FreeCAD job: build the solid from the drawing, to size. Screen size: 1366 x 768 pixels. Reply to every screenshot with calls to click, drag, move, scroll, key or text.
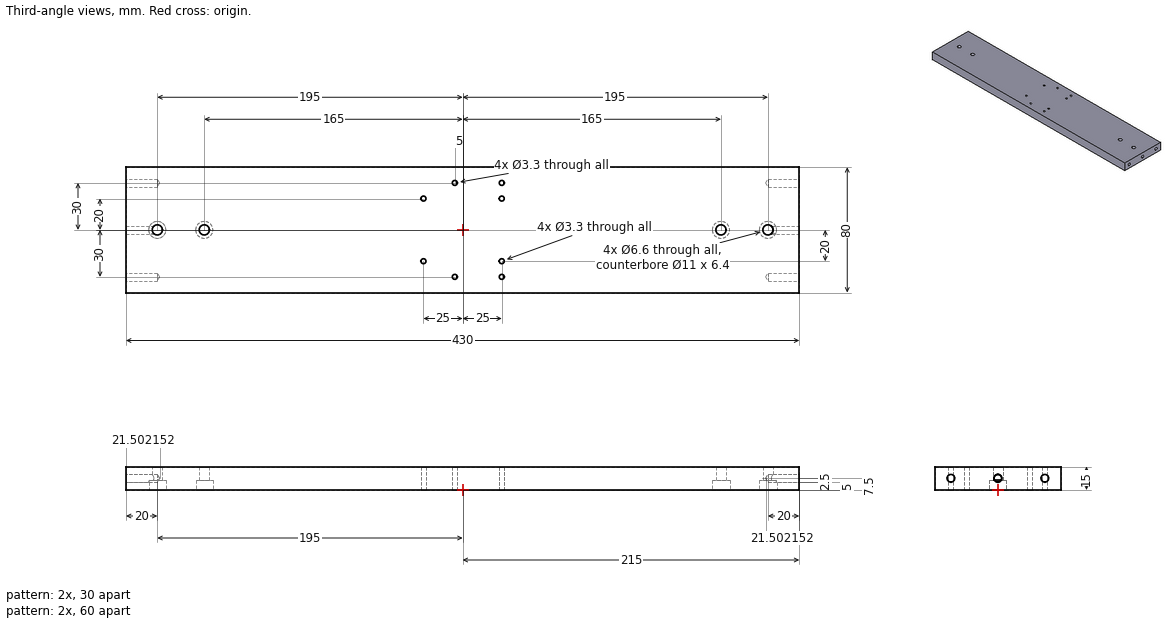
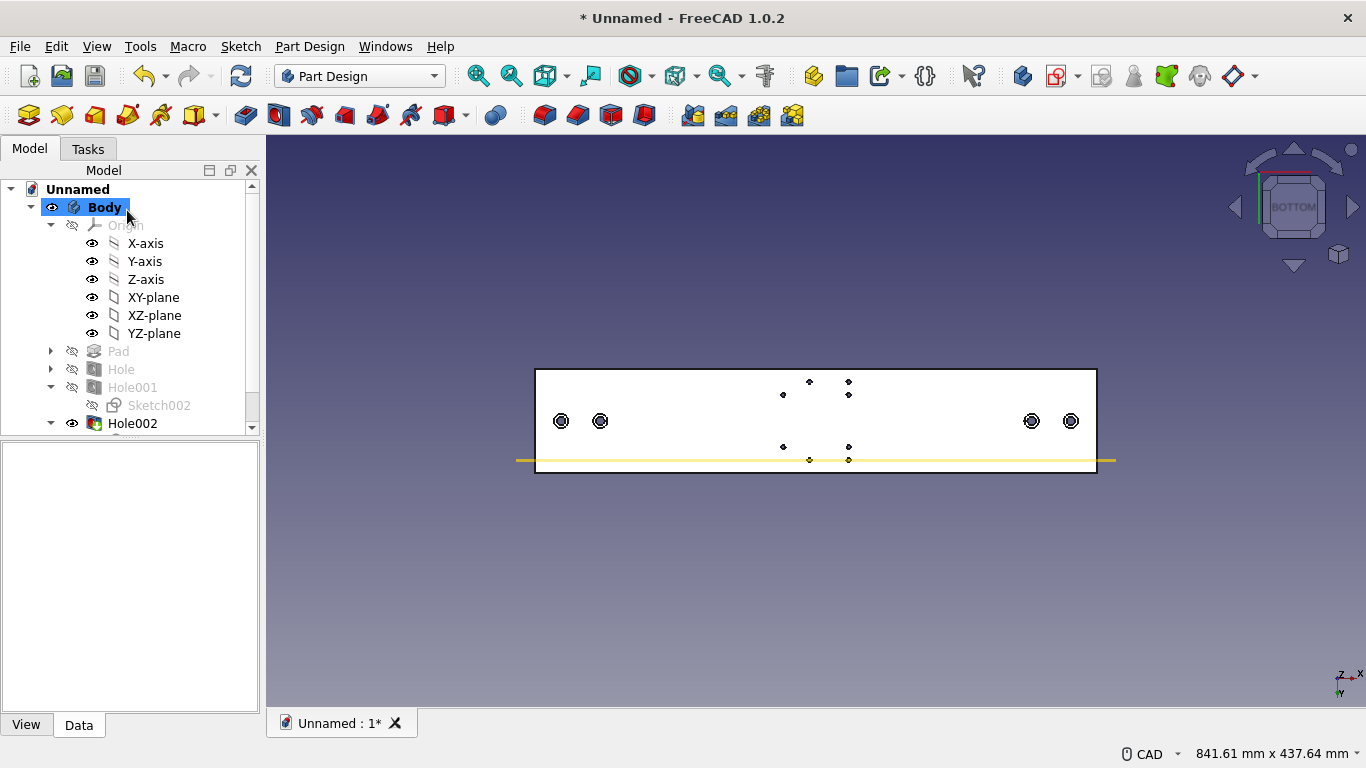
scroll(101, 311, down, 3)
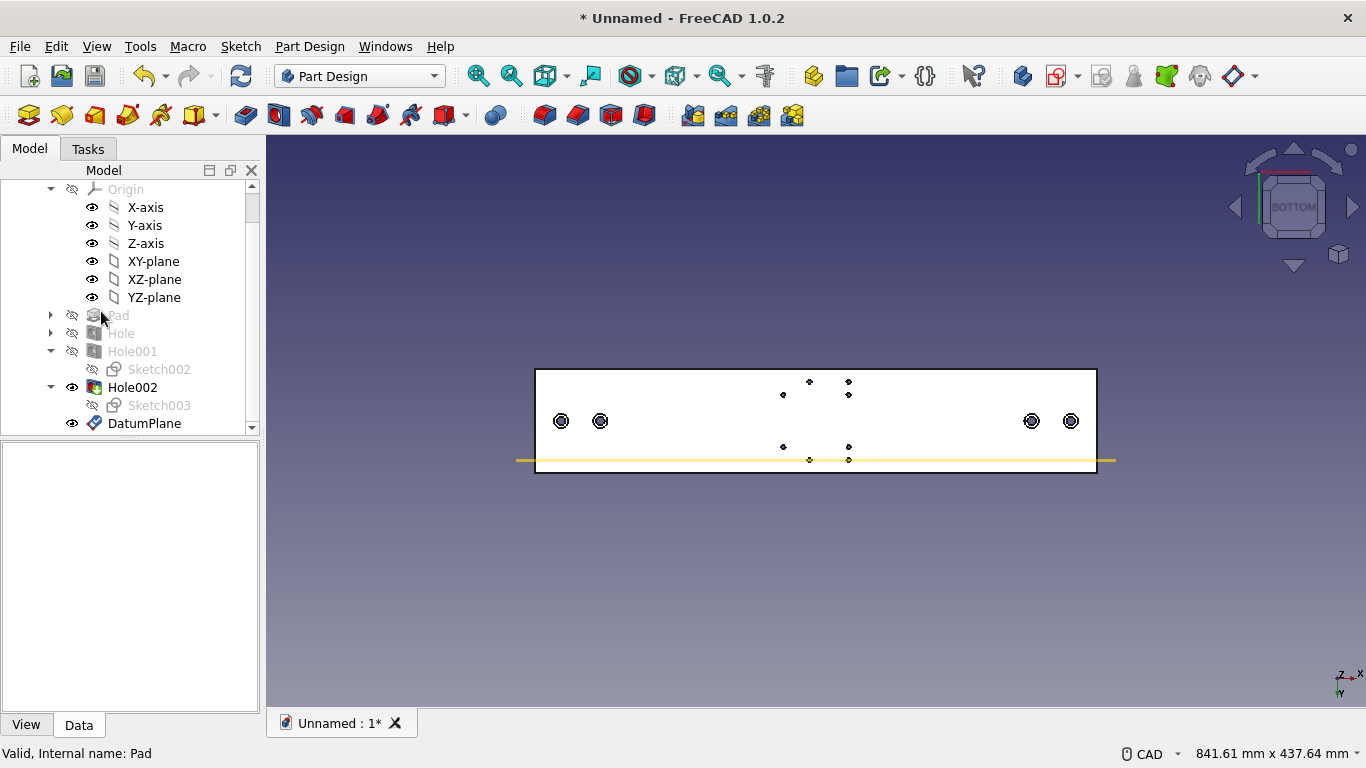
click(117, 423)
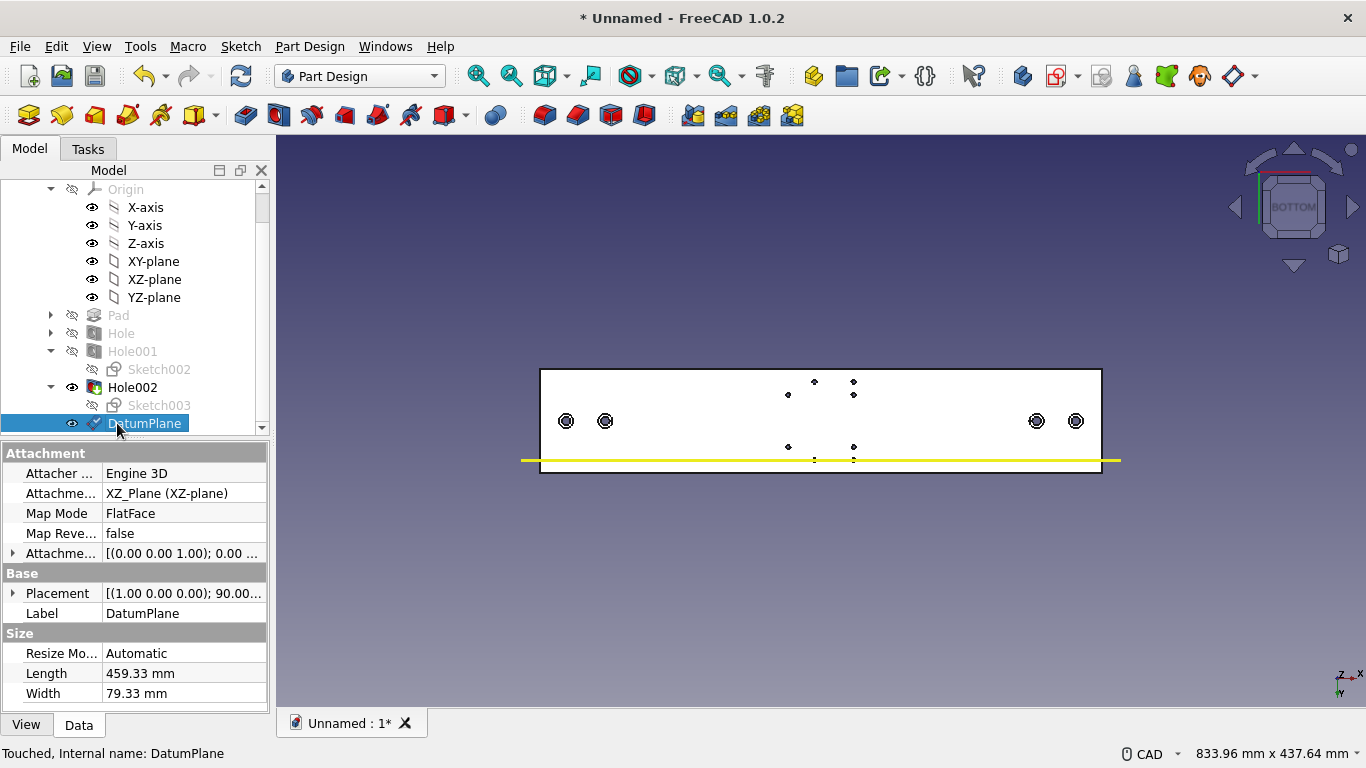
click(1056, 76)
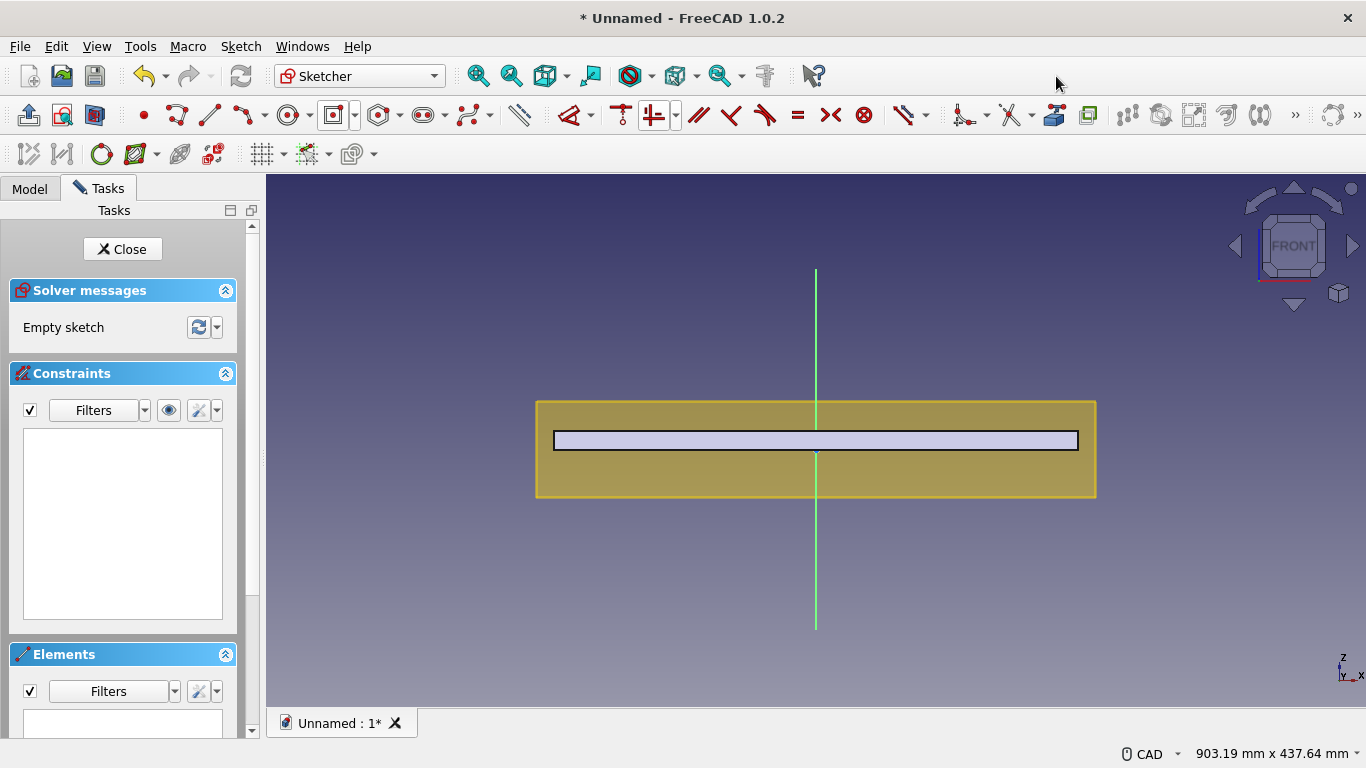
click(95, 116)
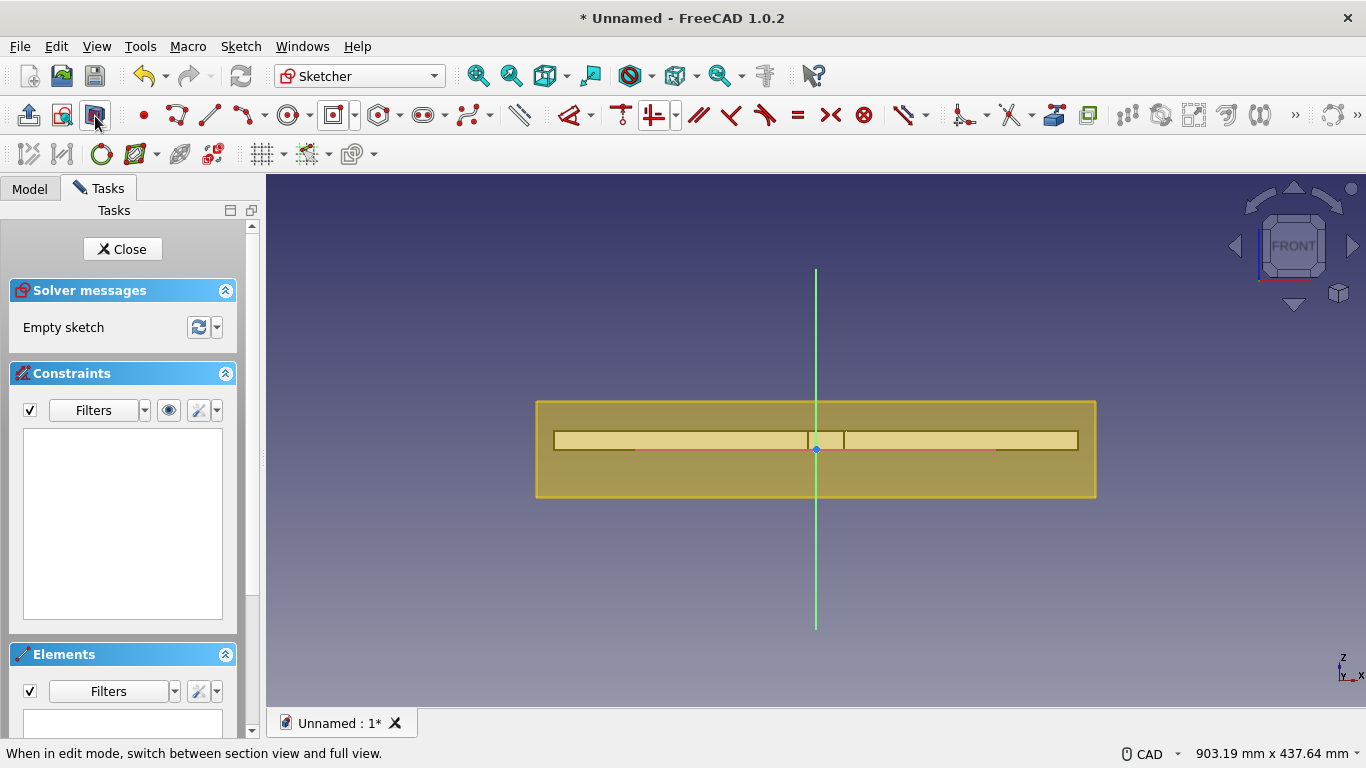
scroll(1080, 442, up, 14)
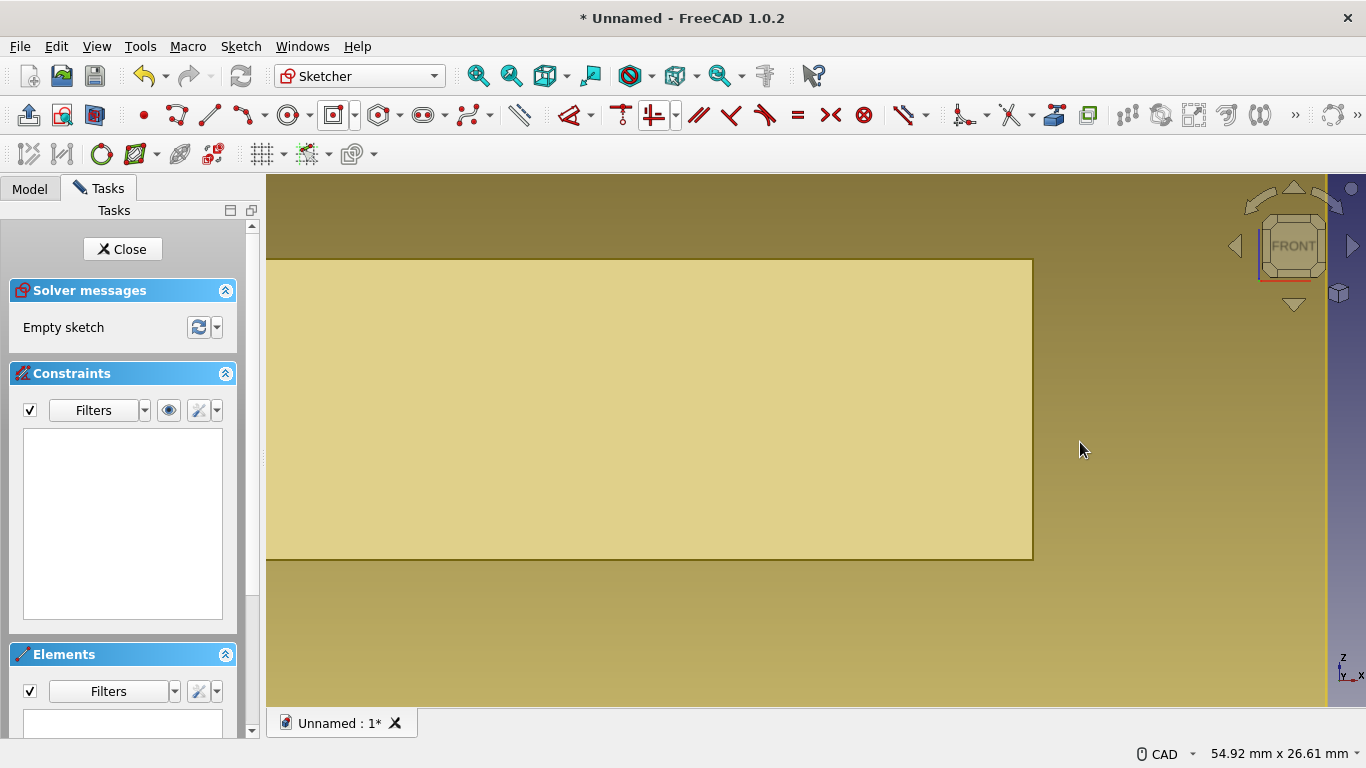
click(177, 116)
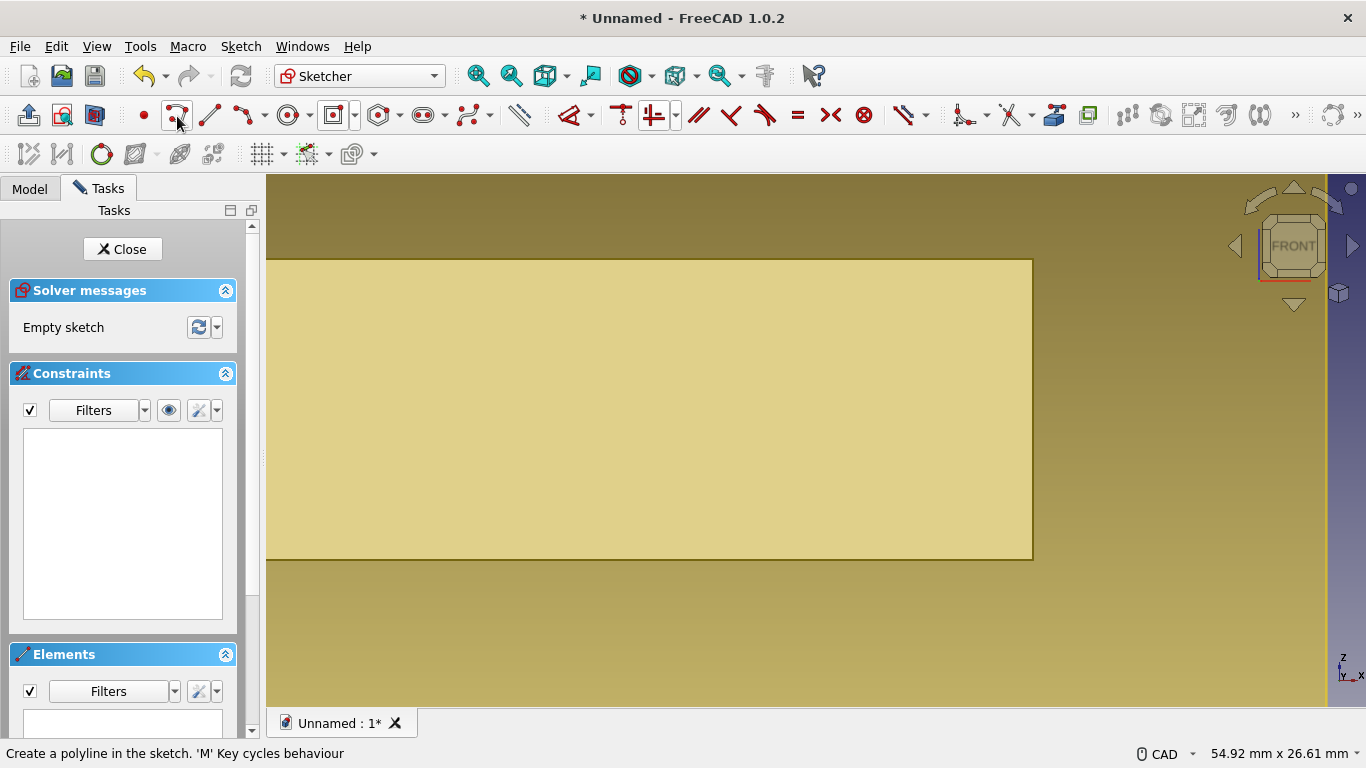
click(603, 410)
click(1033, 410)
click(1033, 460)
click(633, 460)
click(603, 411)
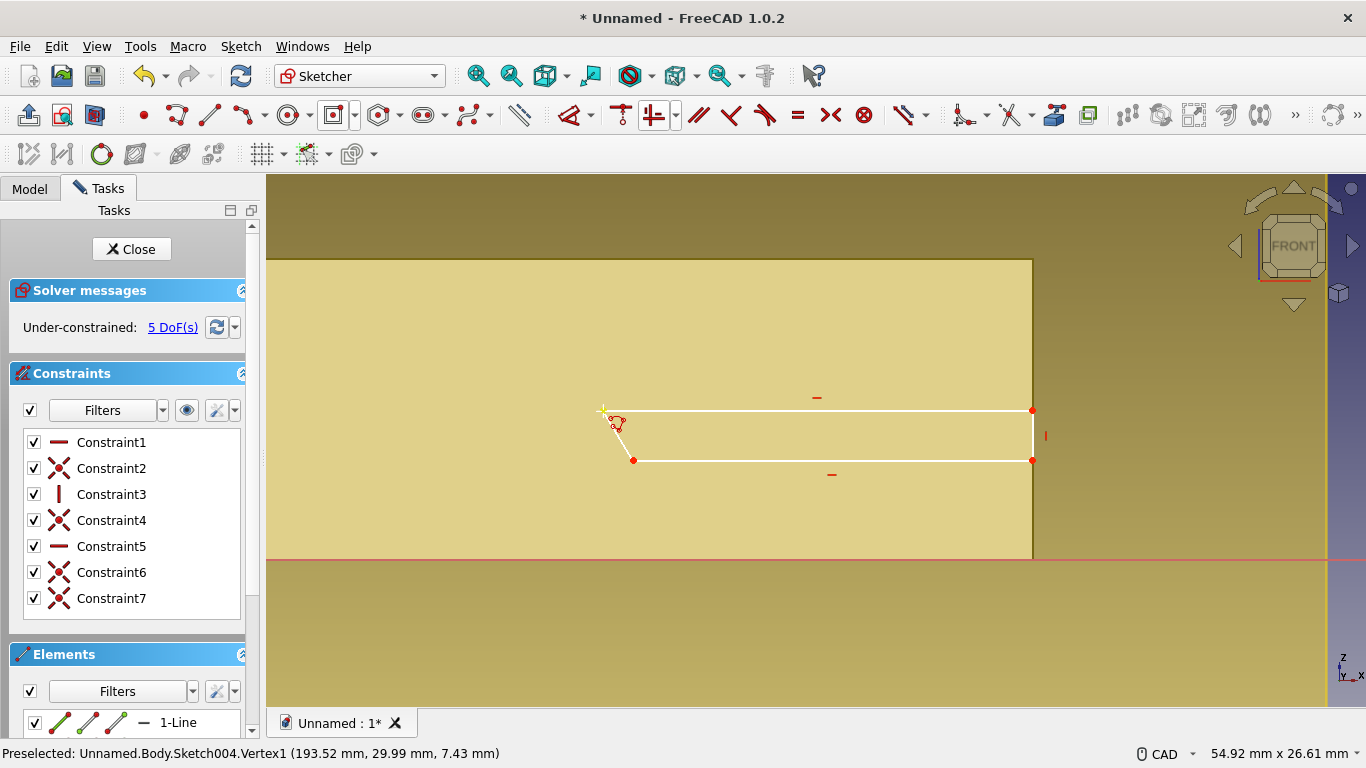
click(210, 116)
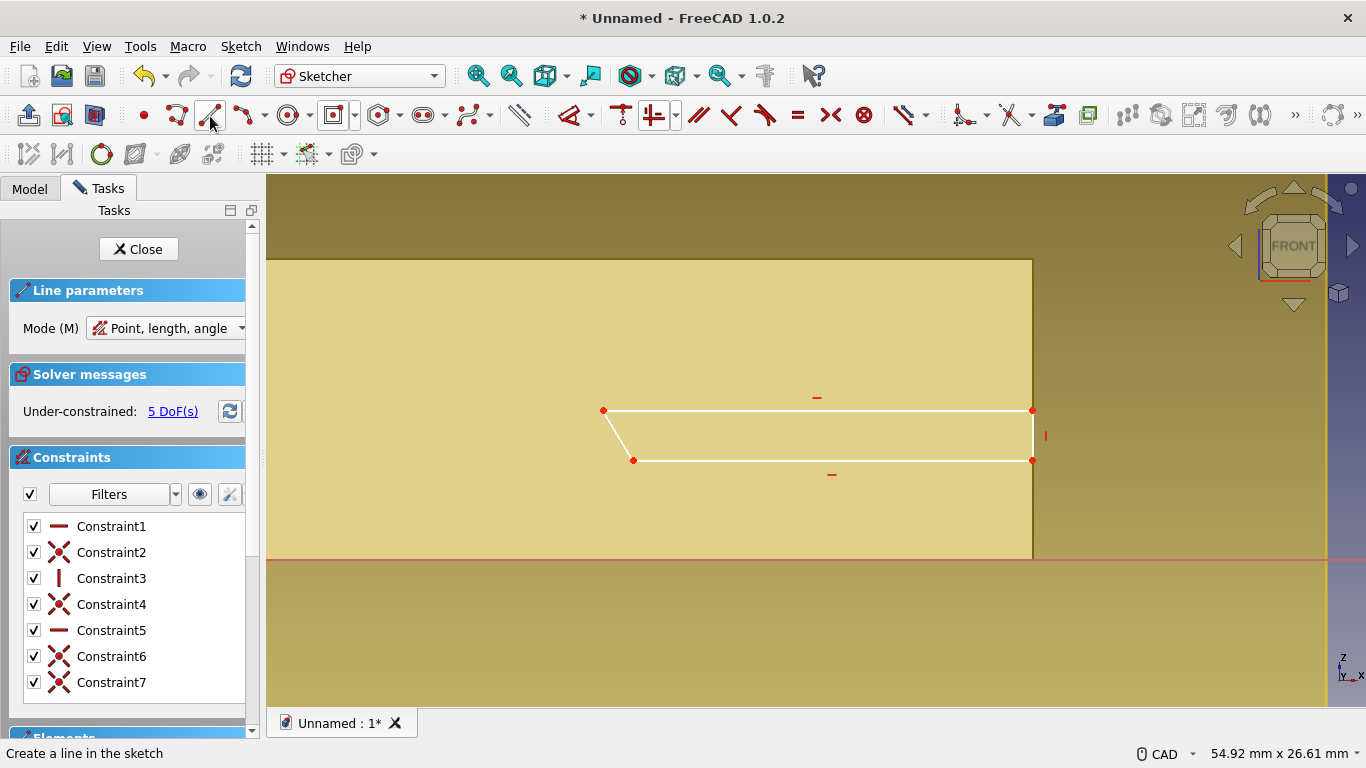
click(559, 410)
click(430, 410)
key(Escape)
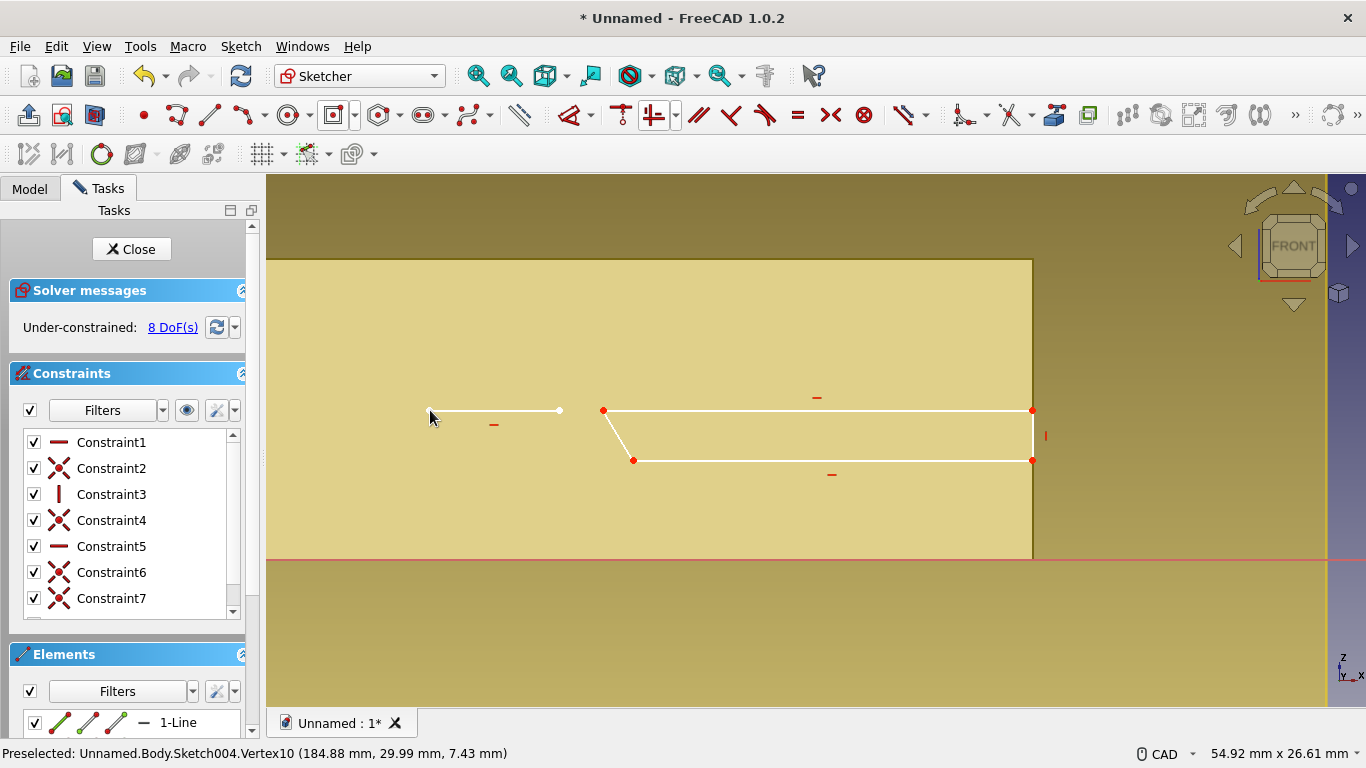
click(520, 411)